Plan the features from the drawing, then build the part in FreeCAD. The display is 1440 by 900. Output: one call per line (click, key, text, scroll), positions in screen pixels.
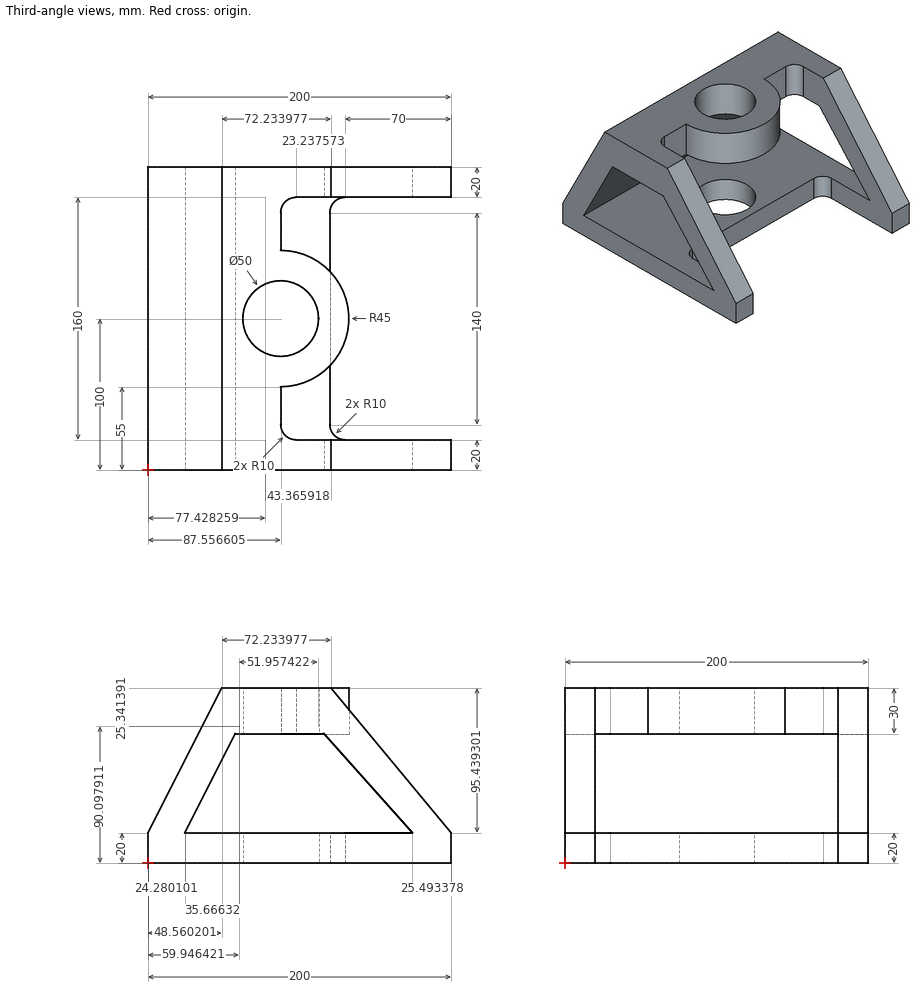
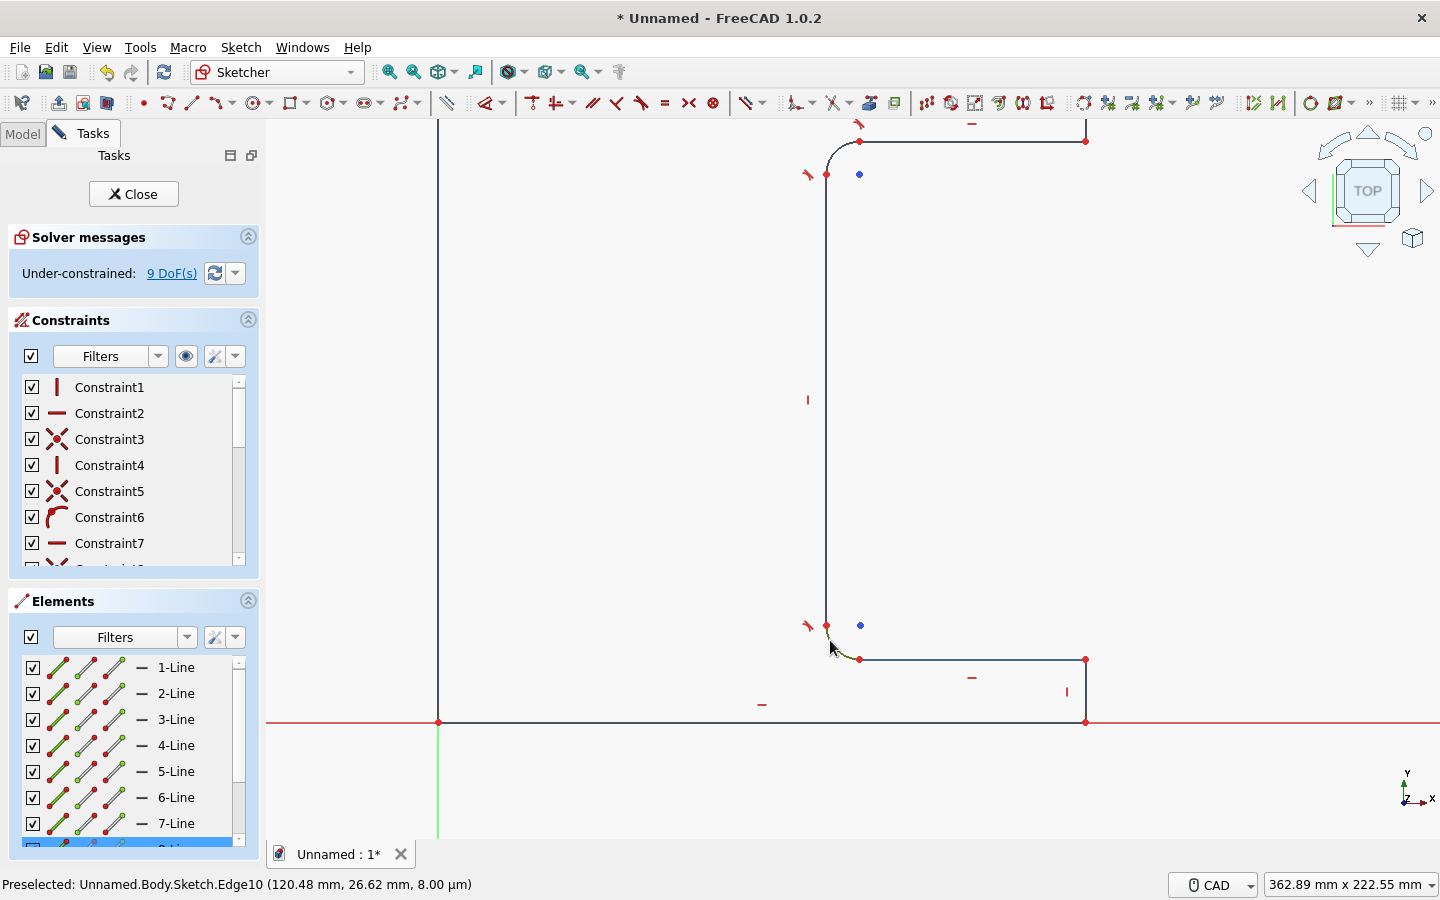
click(642, 104)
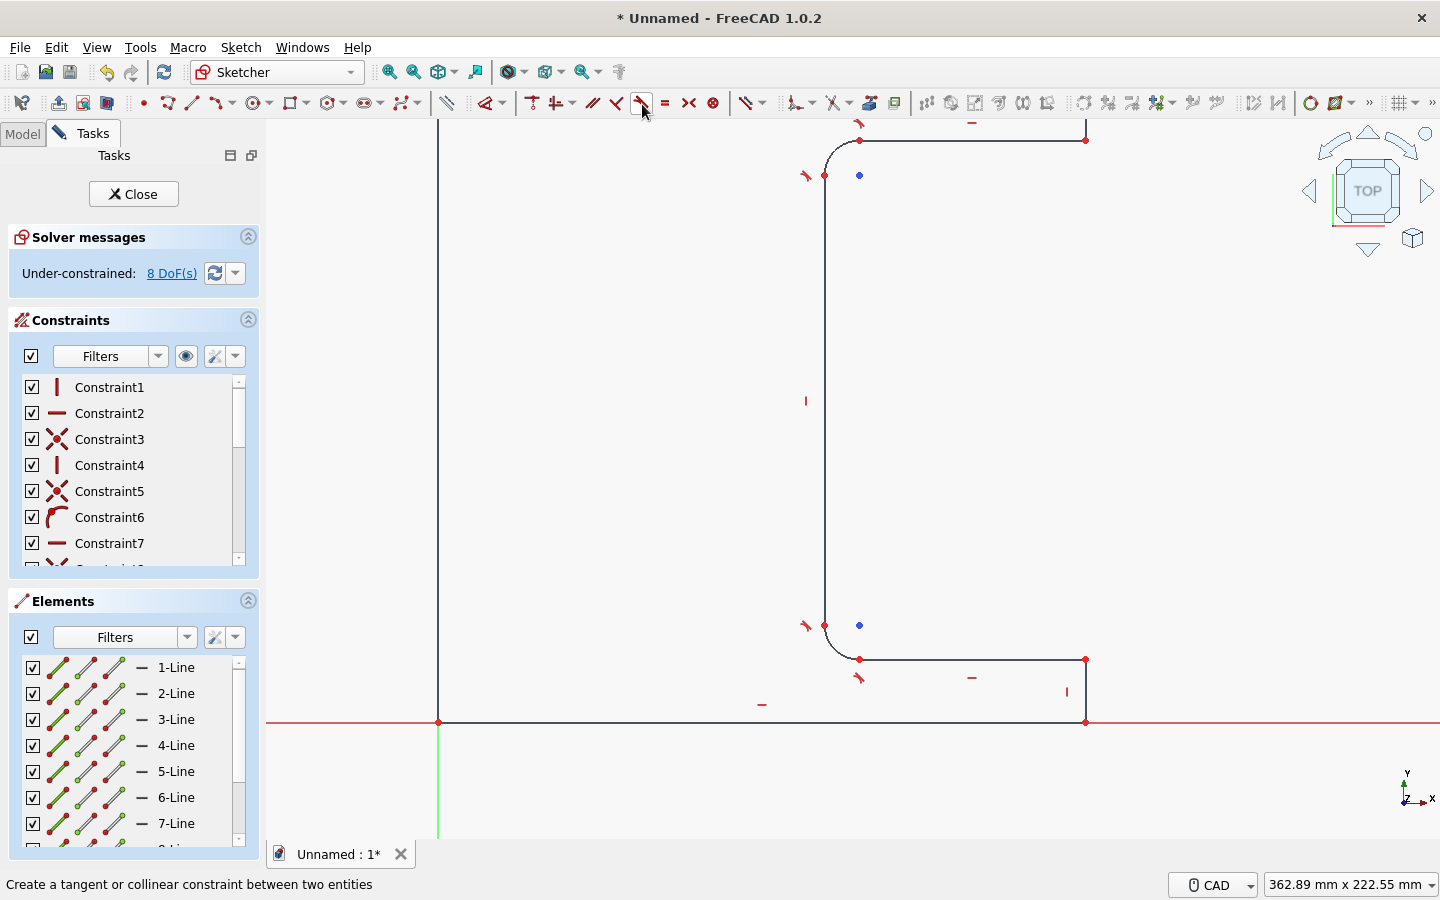
click(828, 160)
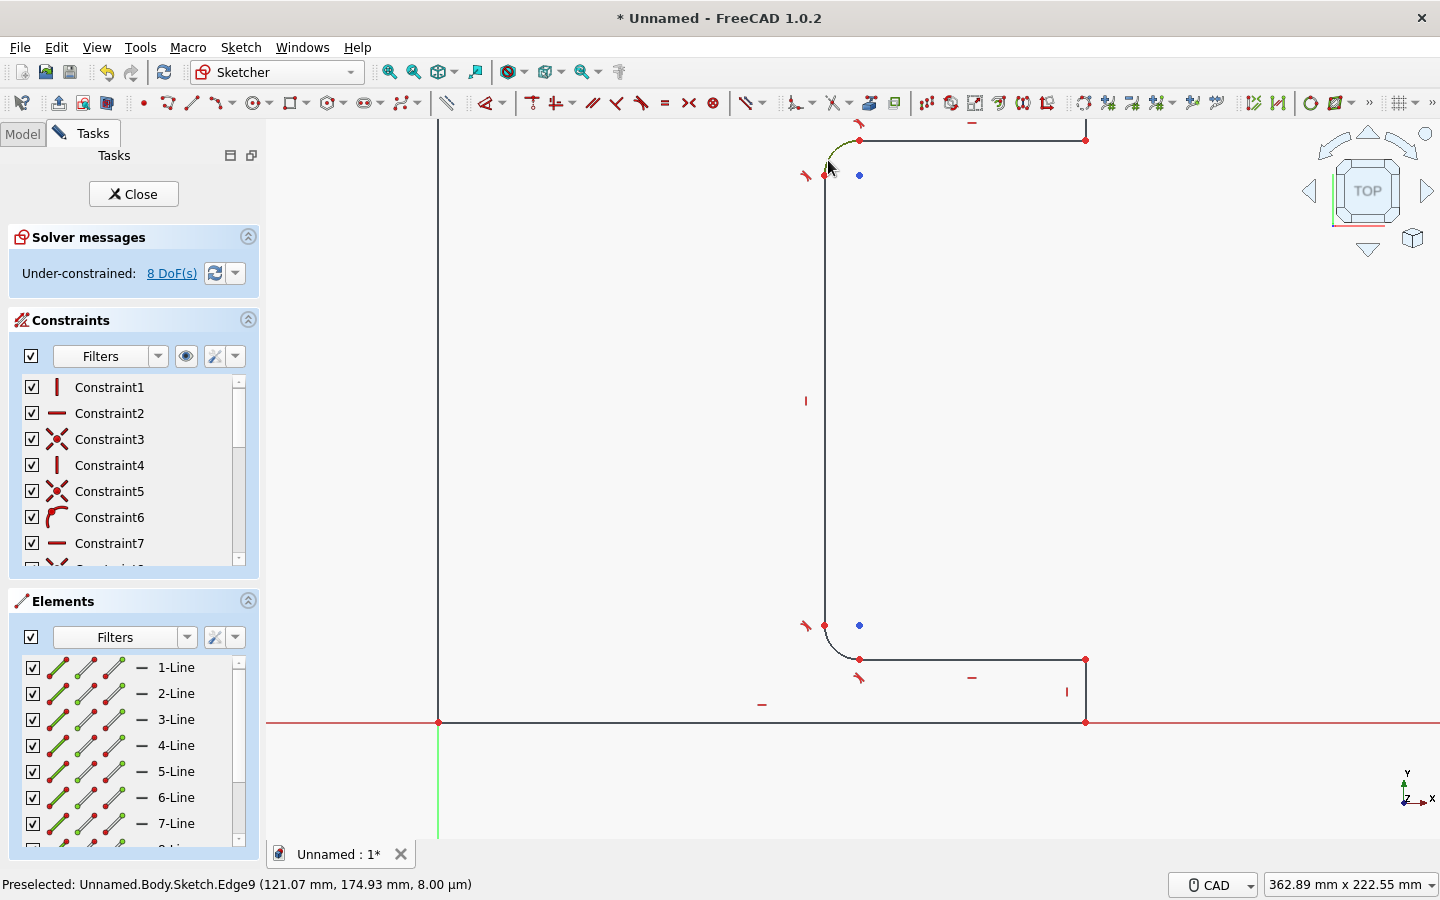
click(828, 641)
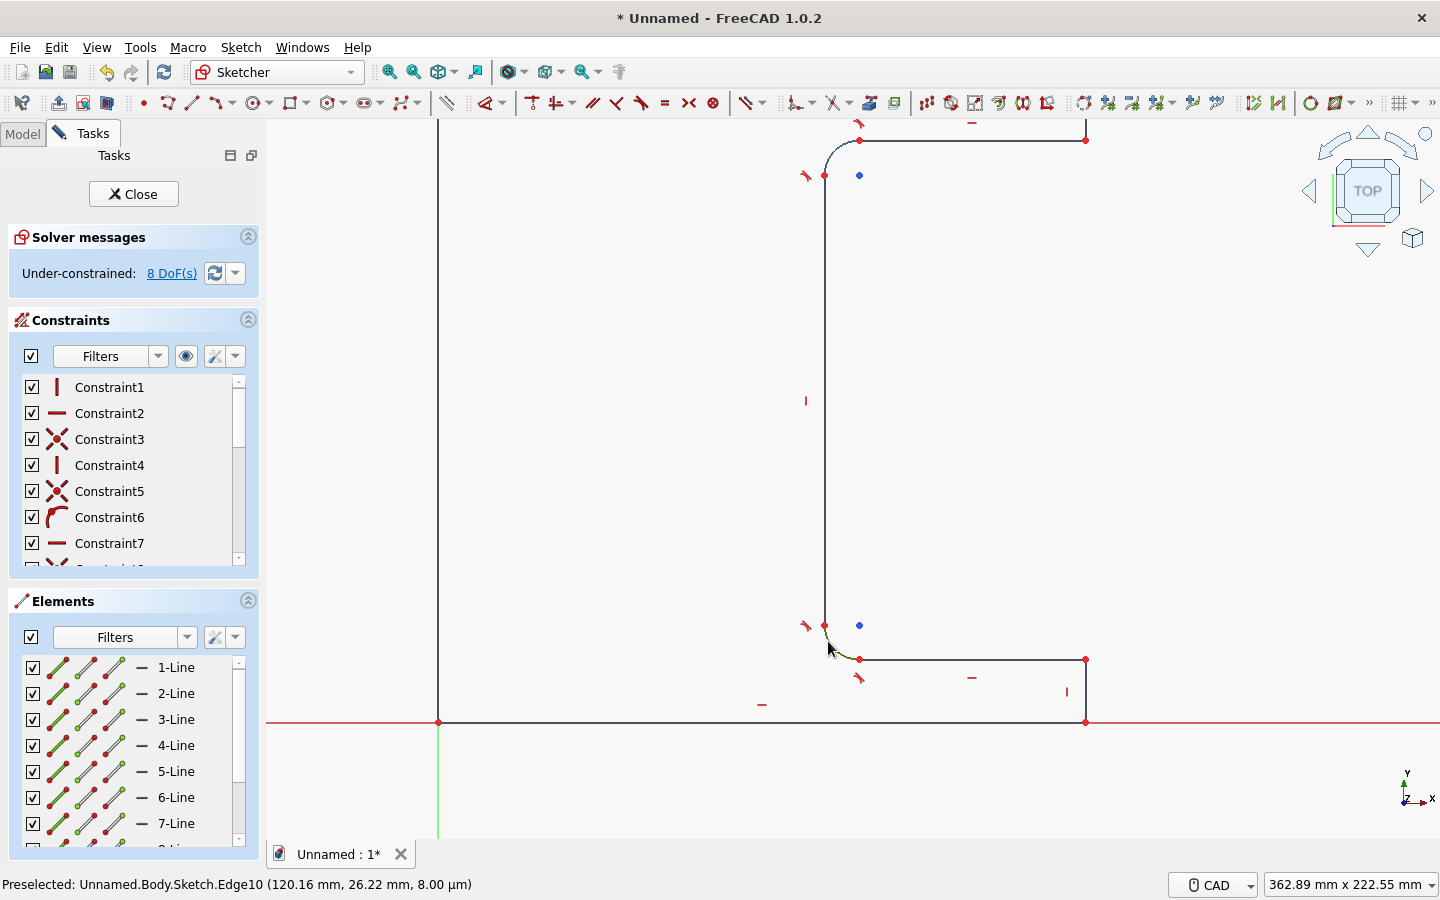
key(e)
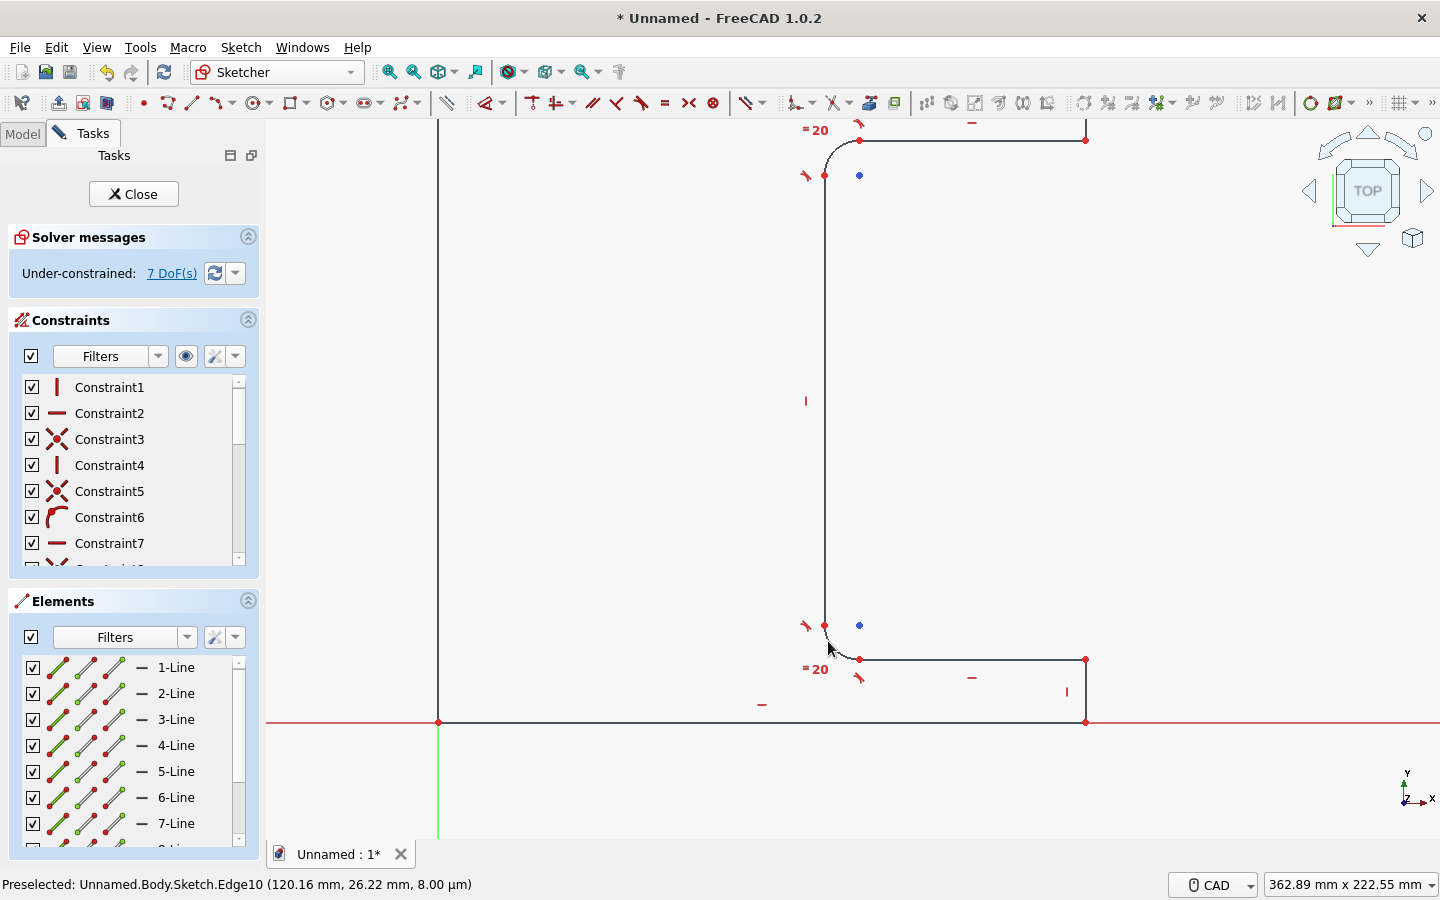
click(486, 104)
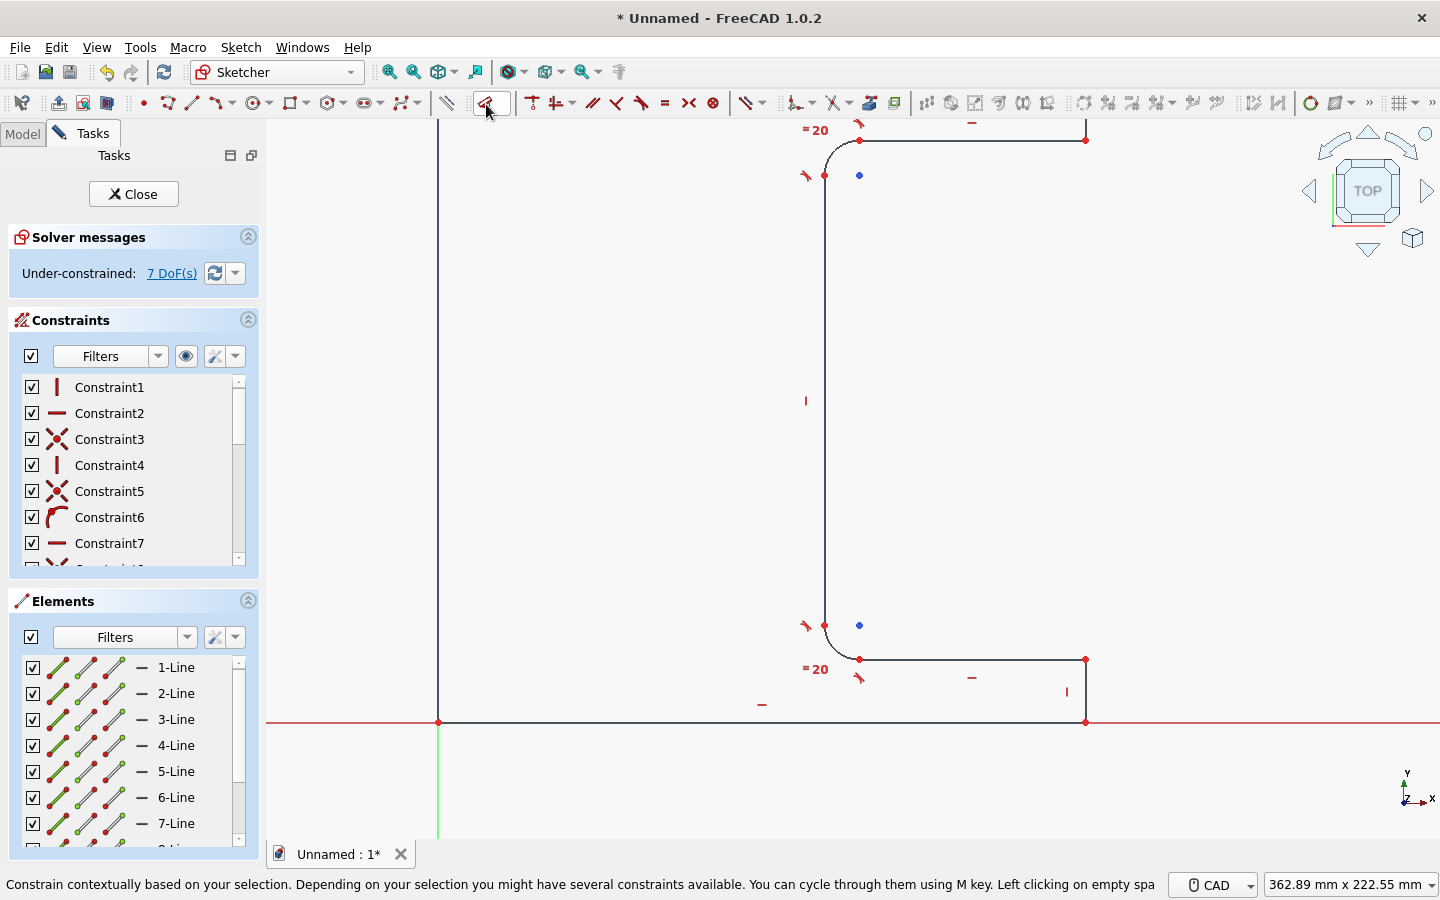
scroll(828, 160, up, 2)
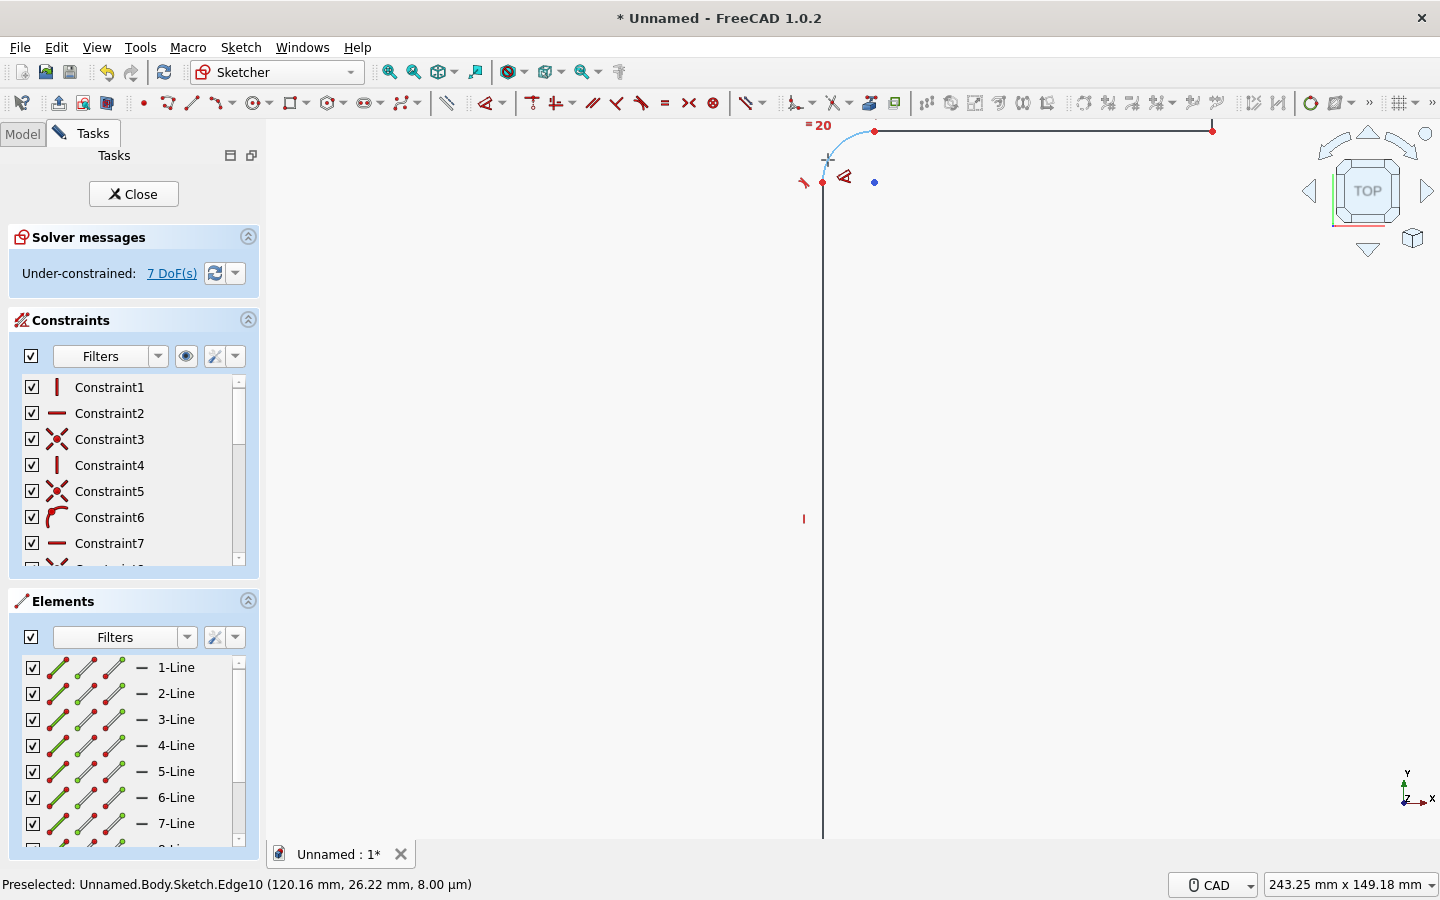
click(828, 159)
click(790, 185)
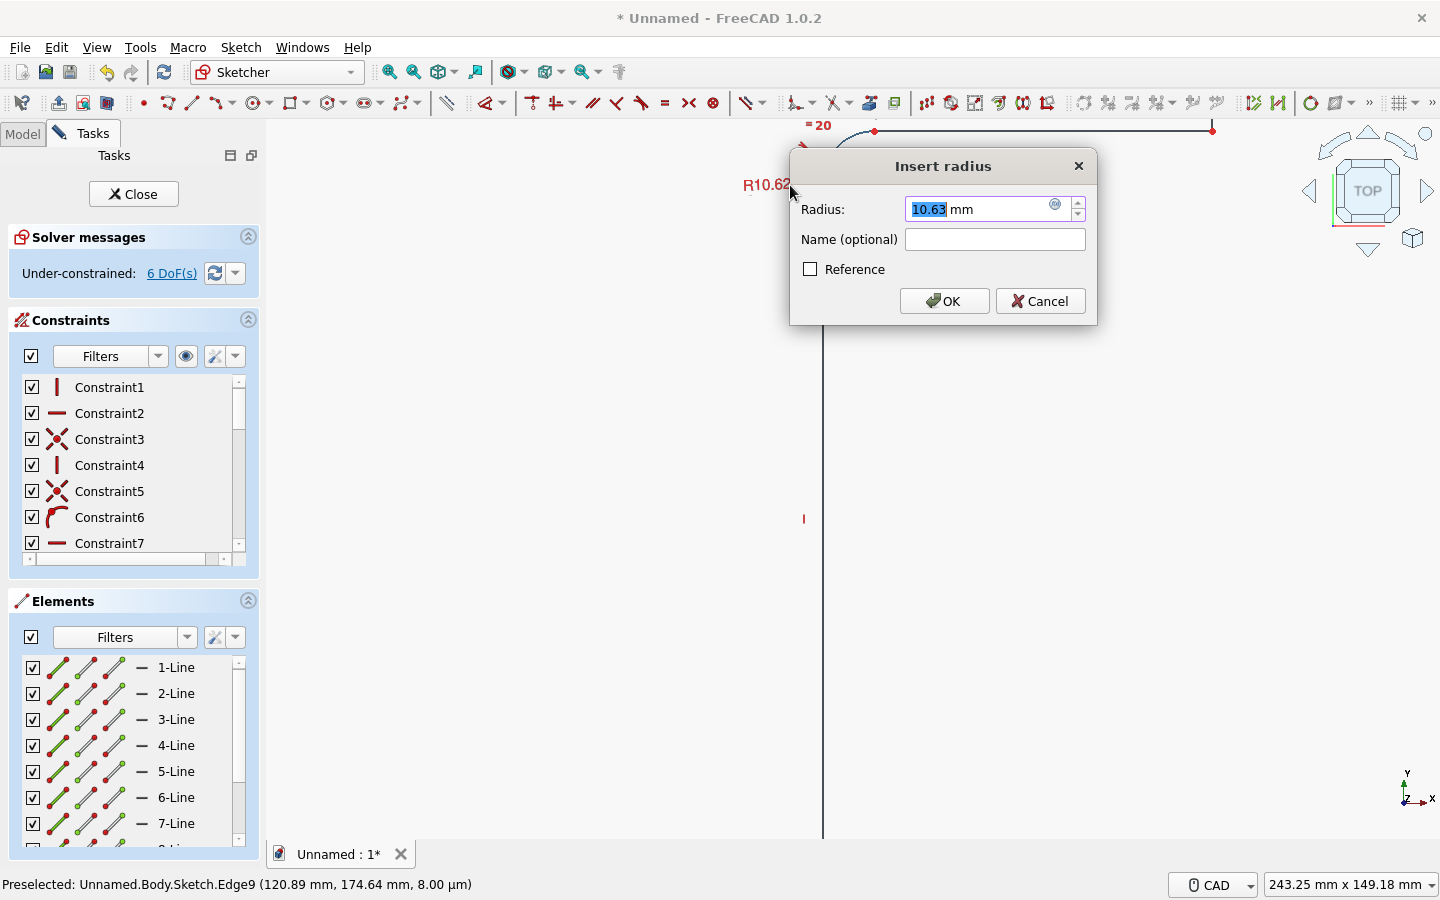
text(10)
key(Return)